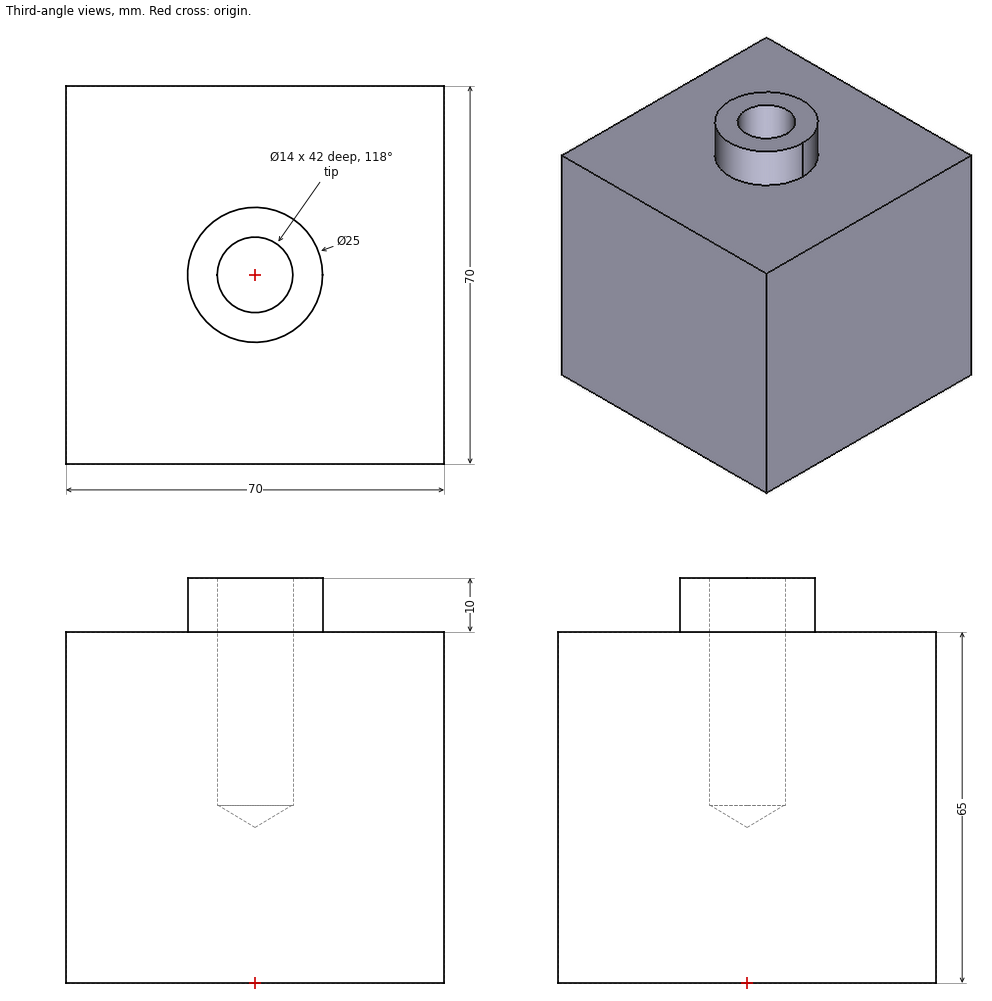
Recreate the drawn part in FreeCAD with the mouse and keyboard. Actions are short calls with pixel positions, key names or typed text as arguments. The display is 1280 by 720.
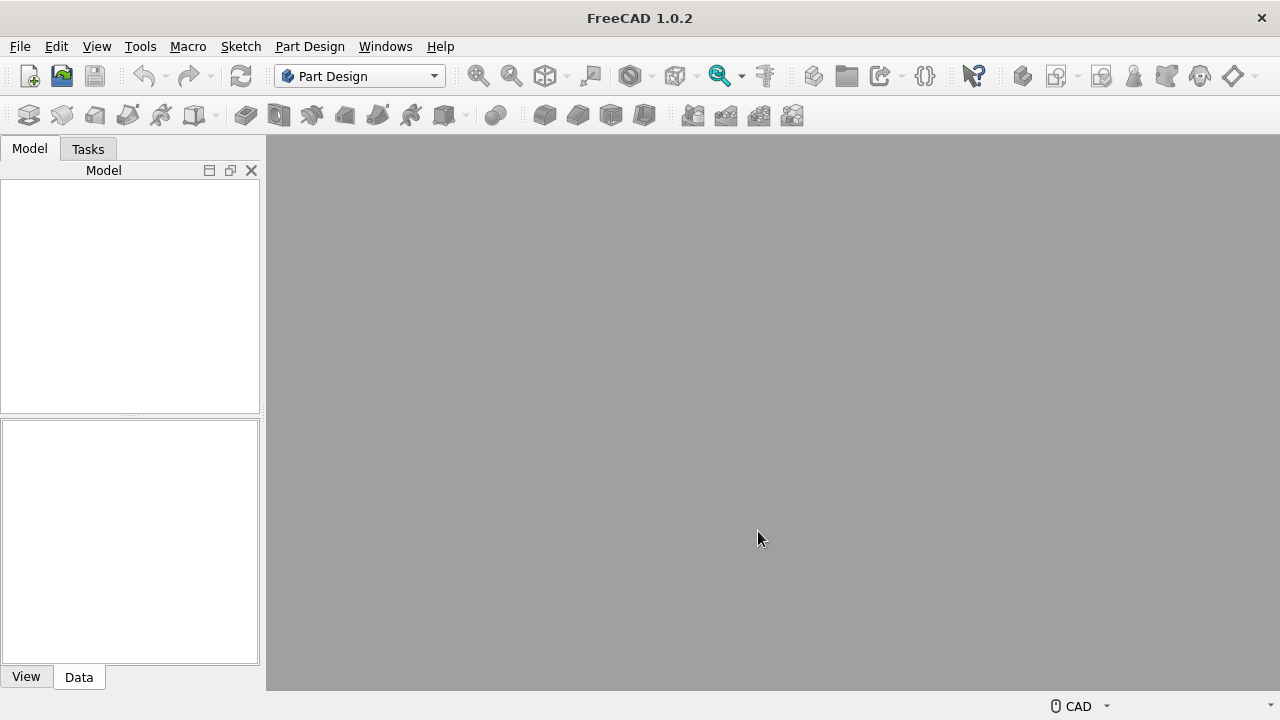
click(29, 76)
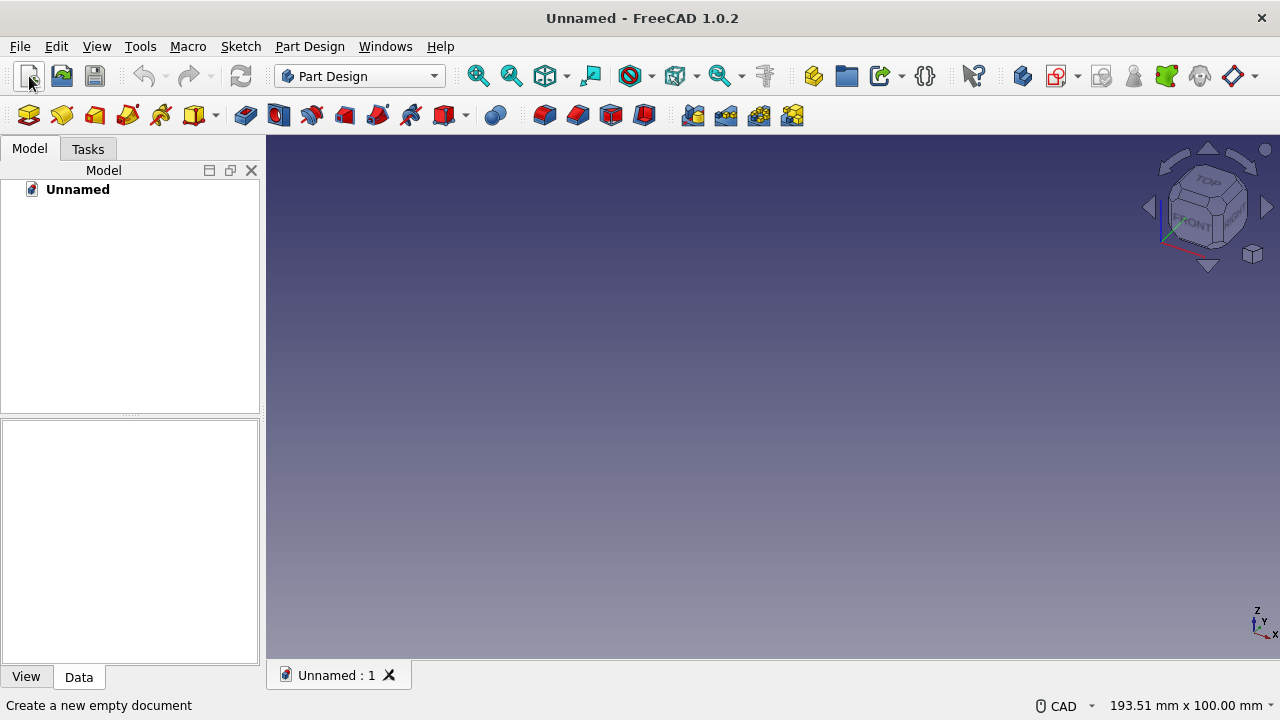
click(1056, 76)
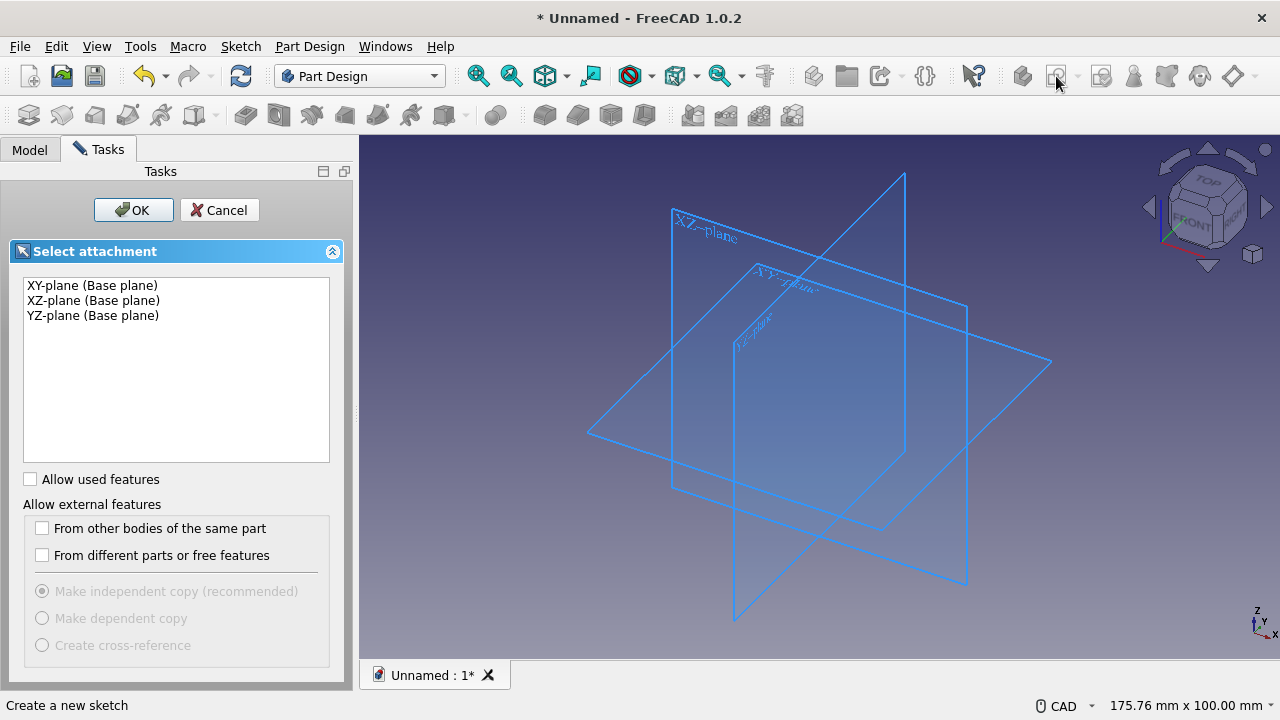
click(84, 286)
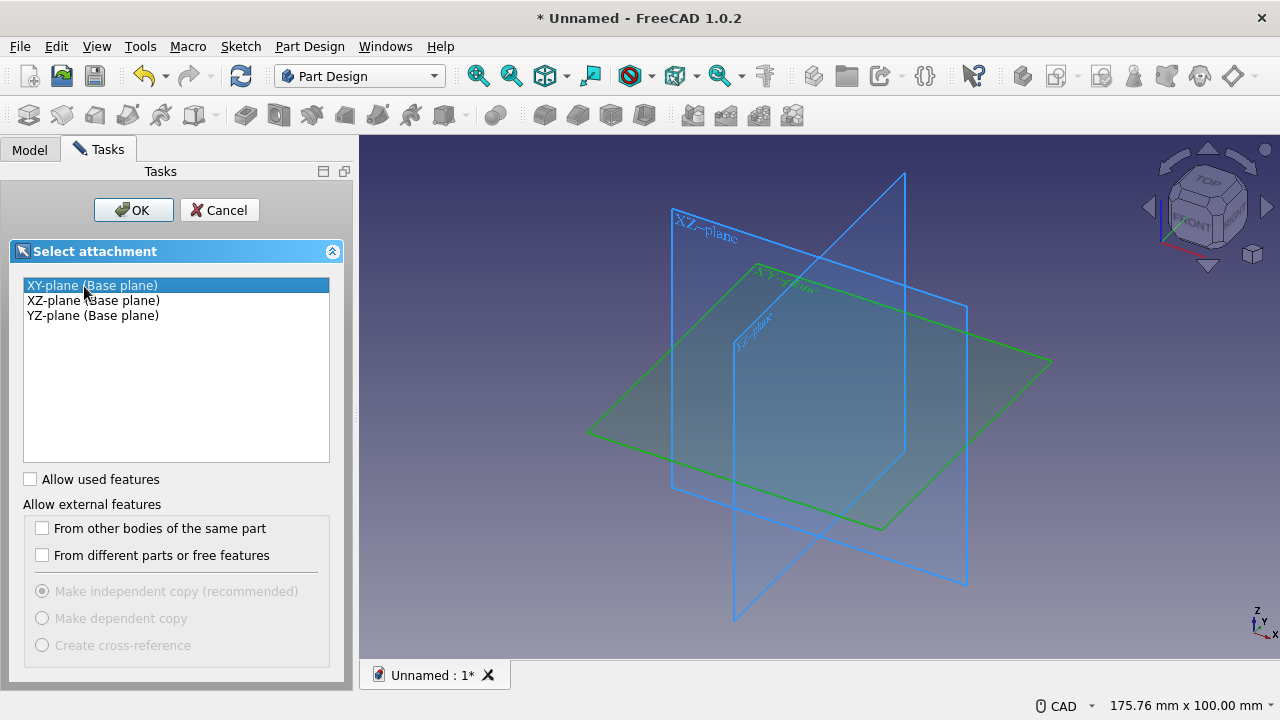
click(134, 210)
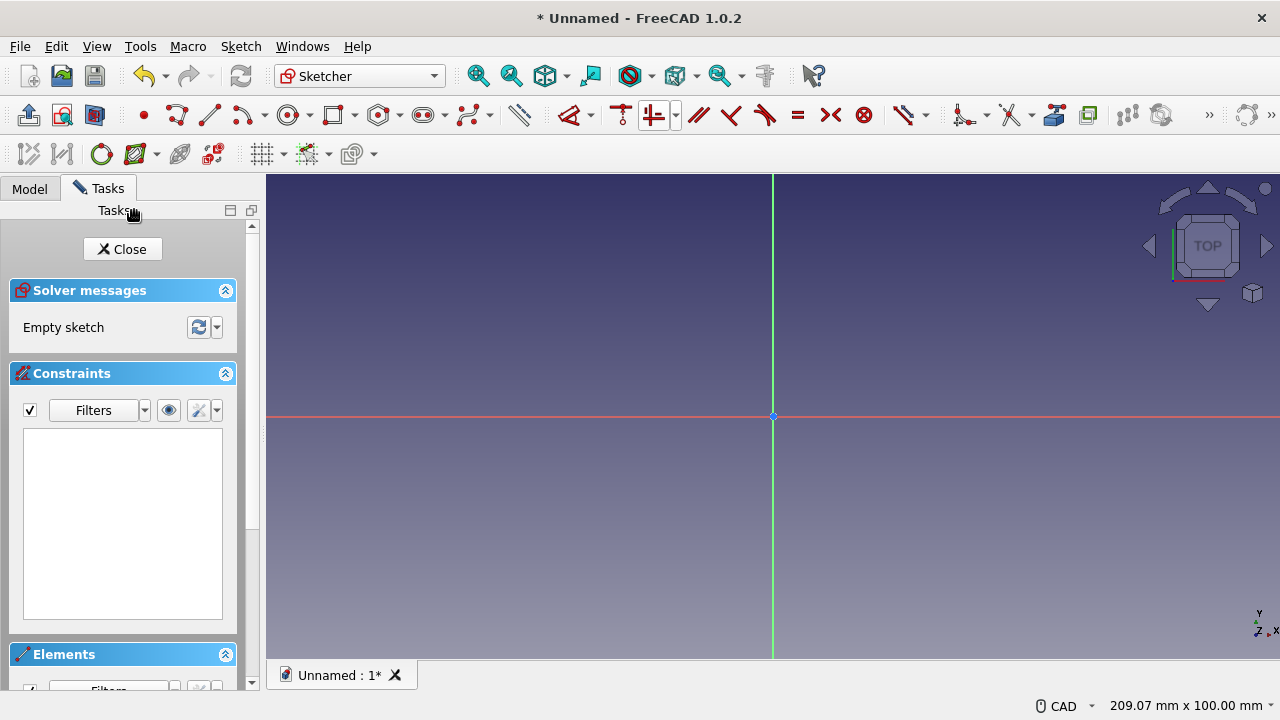
key(g)
key(v)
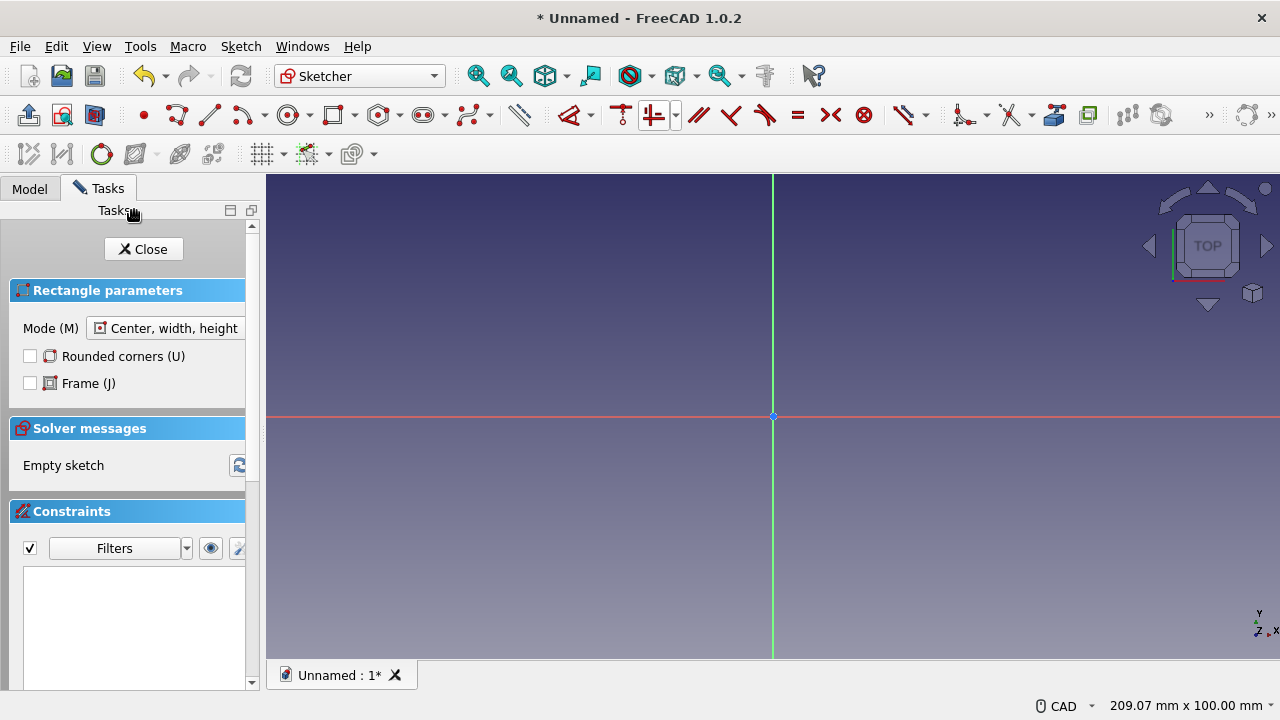
click(773, 416)
click(943, 247)
key(Escape)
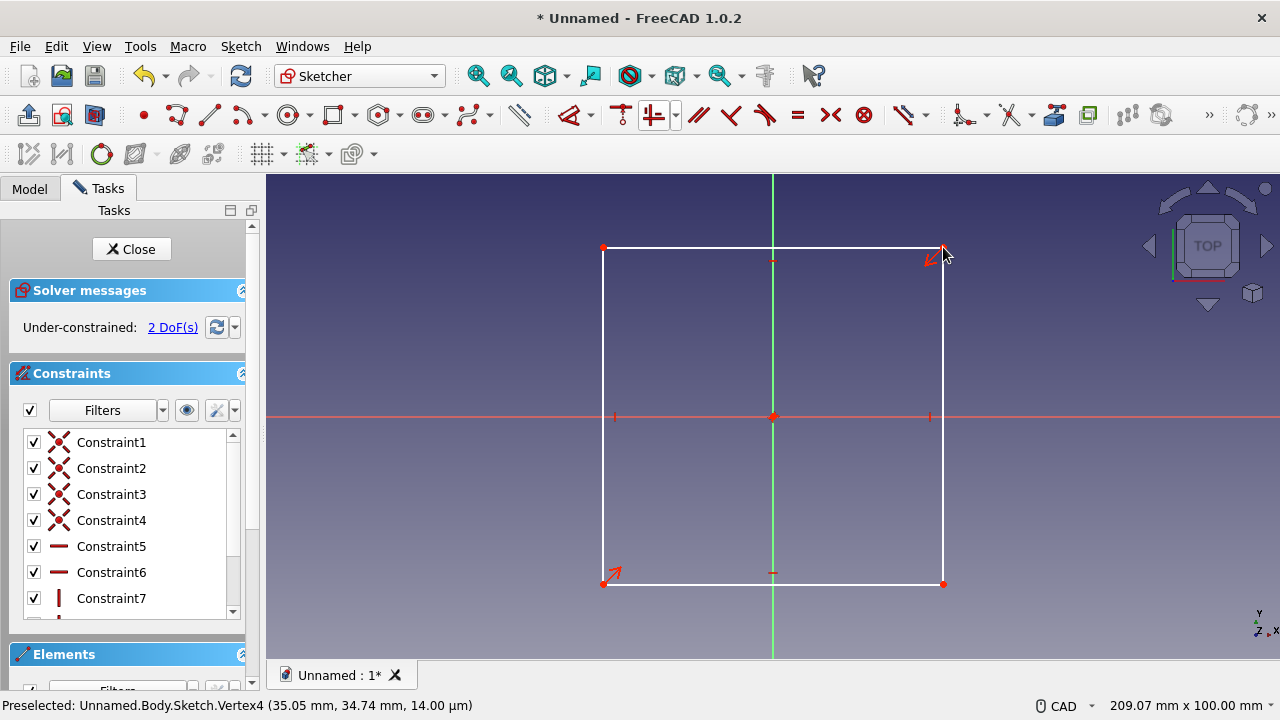
click(568, 116)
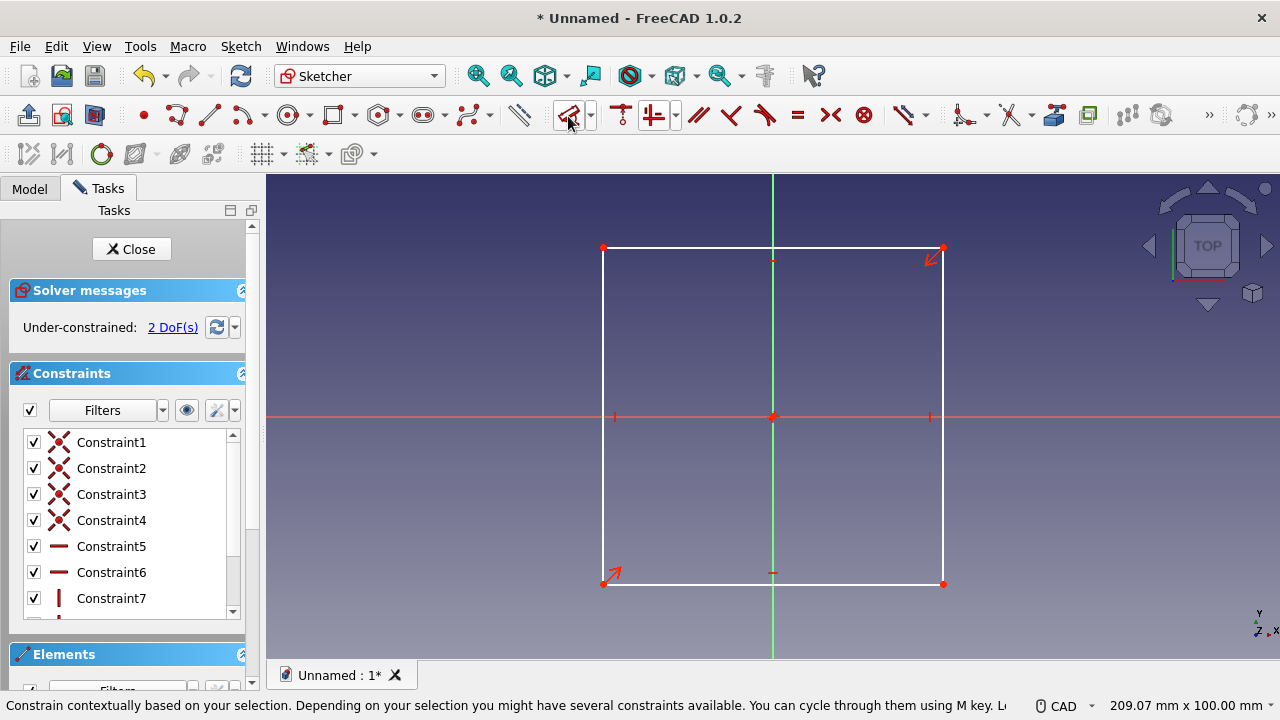
click(705, 585)
click(695, 619)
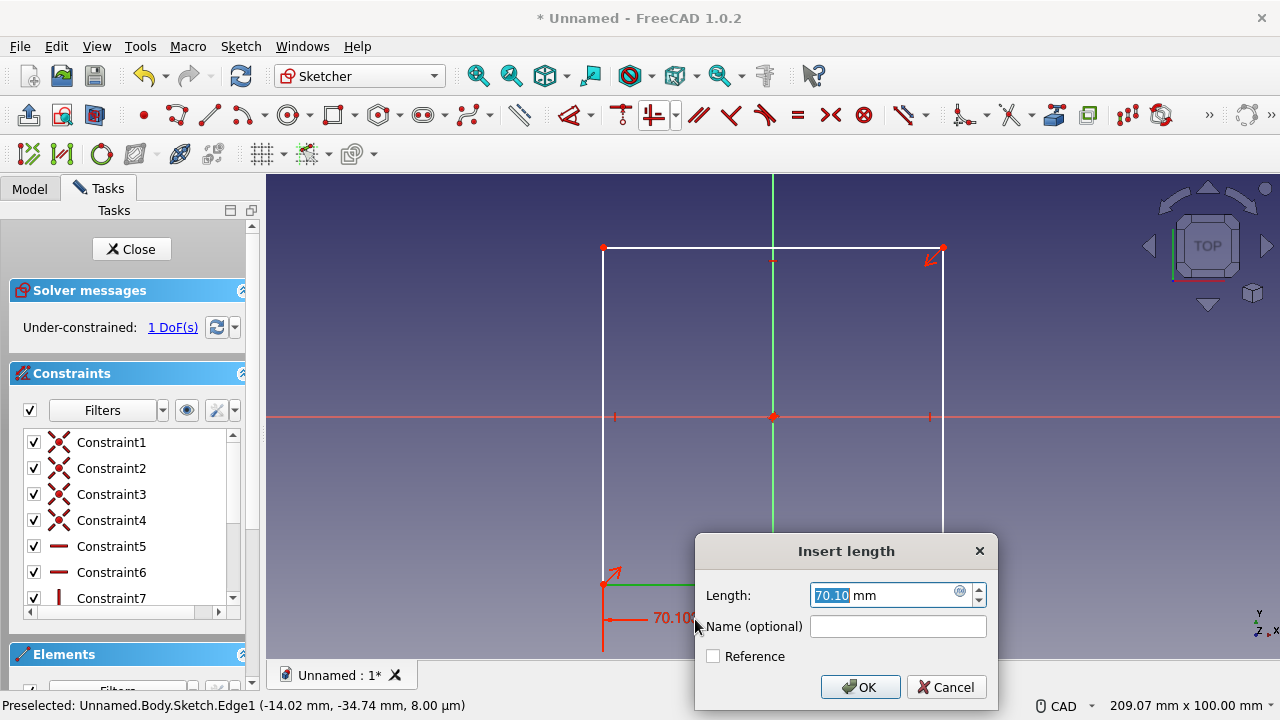
text(70)
key(Return)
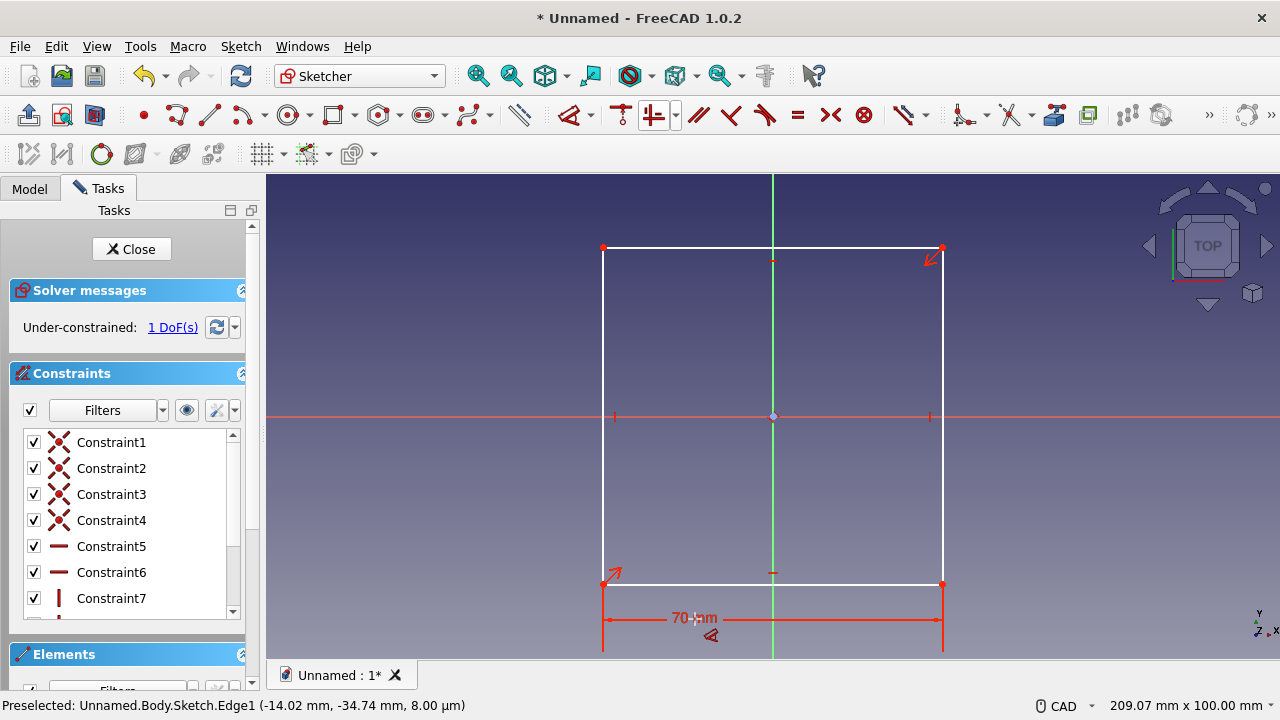
click(943, 484)
click(977, 339)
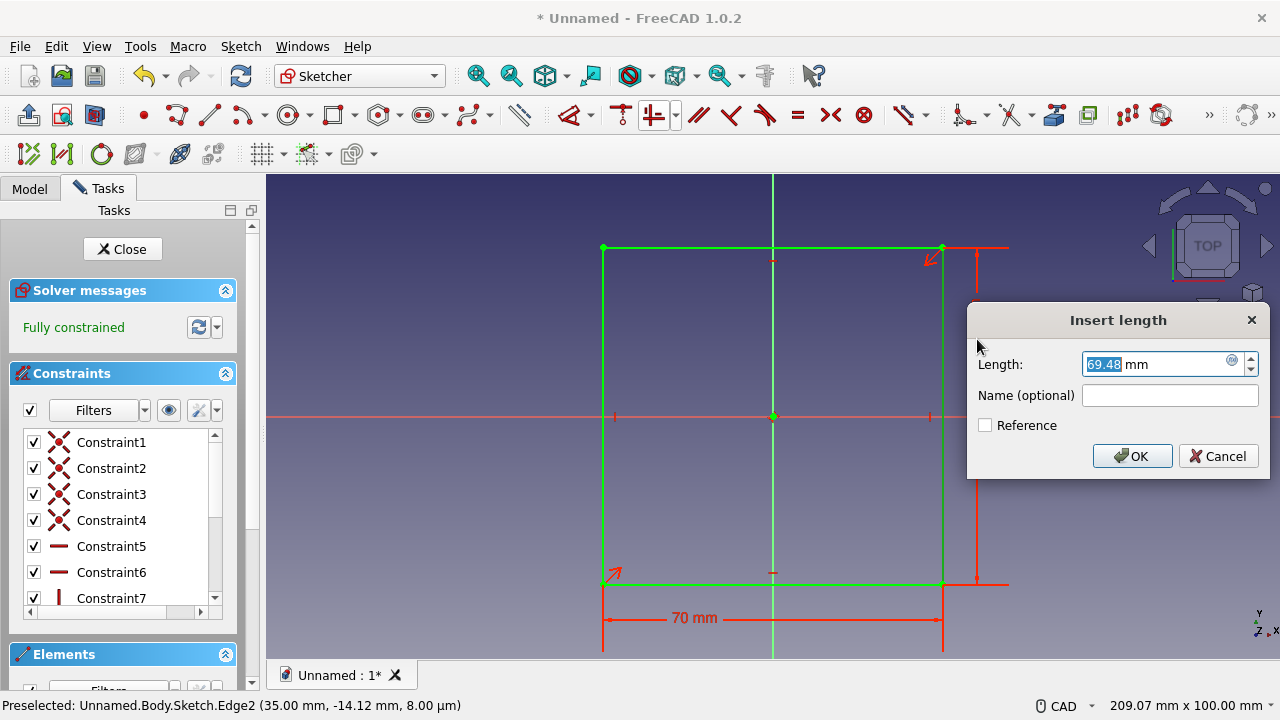
text(70)
key(Return)
key(Escape)